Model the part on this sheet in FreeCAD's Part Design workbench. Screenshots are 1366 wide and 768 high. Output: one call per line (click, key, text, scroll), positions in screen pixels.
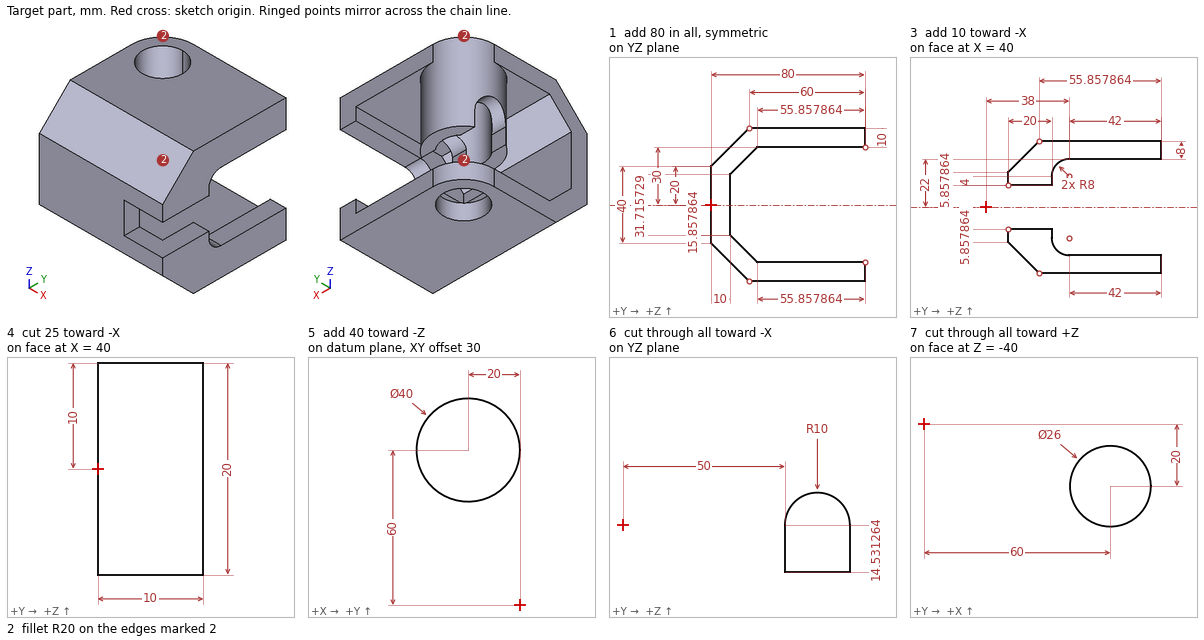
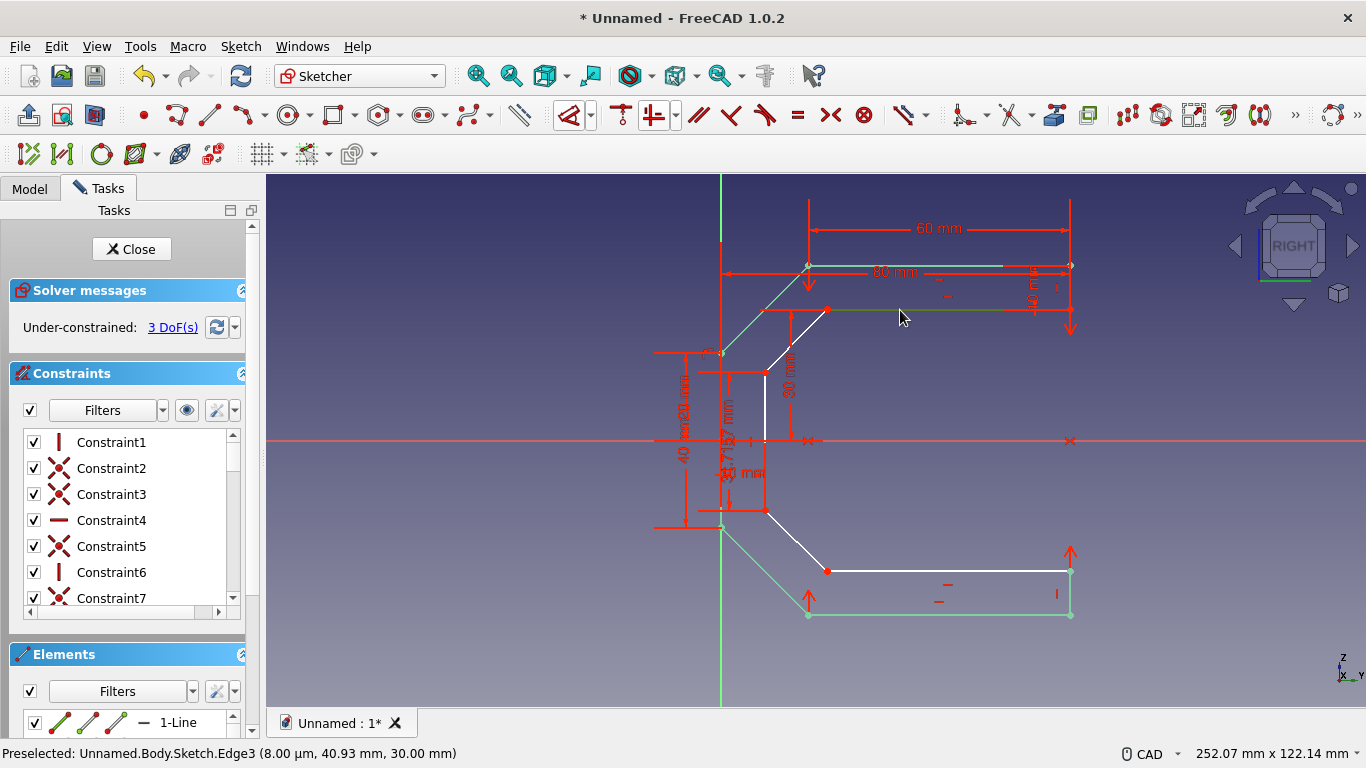
key(l)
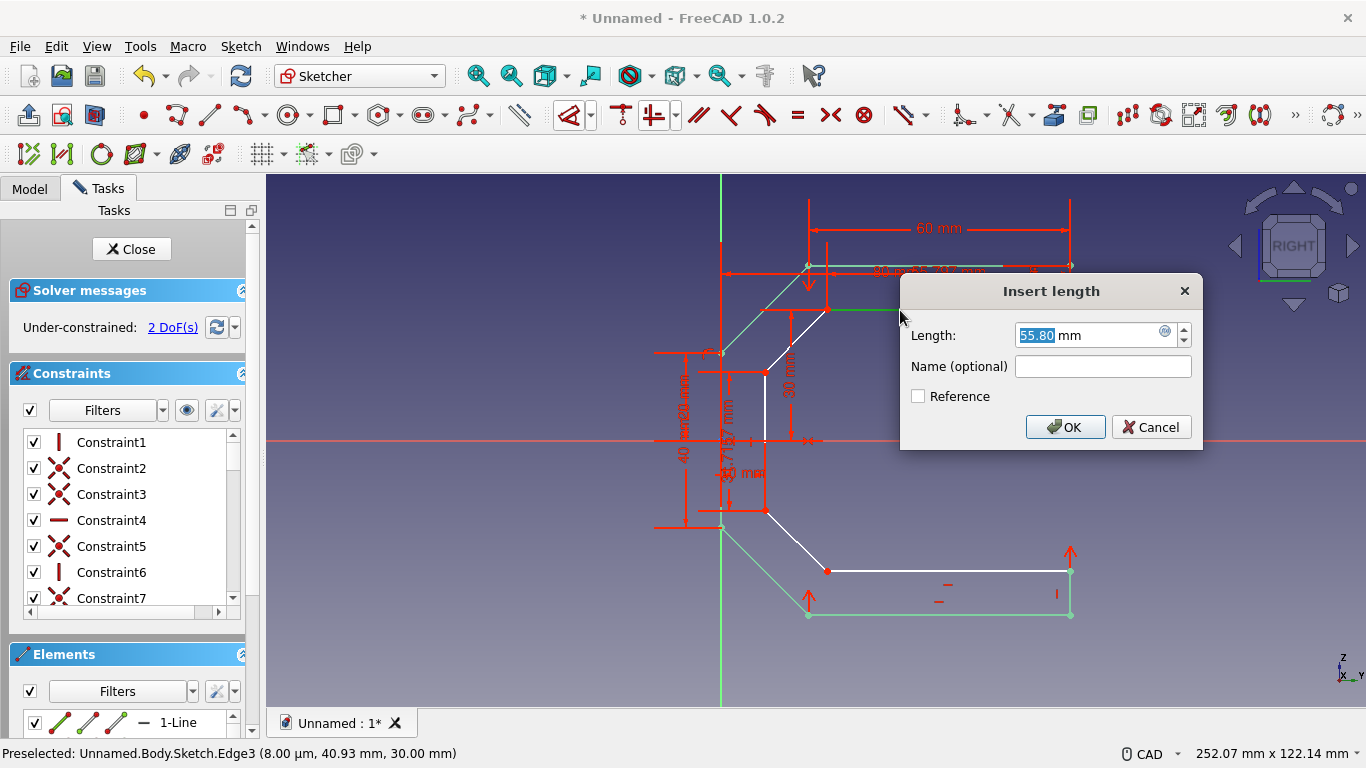
text(55.857864)
key(Return)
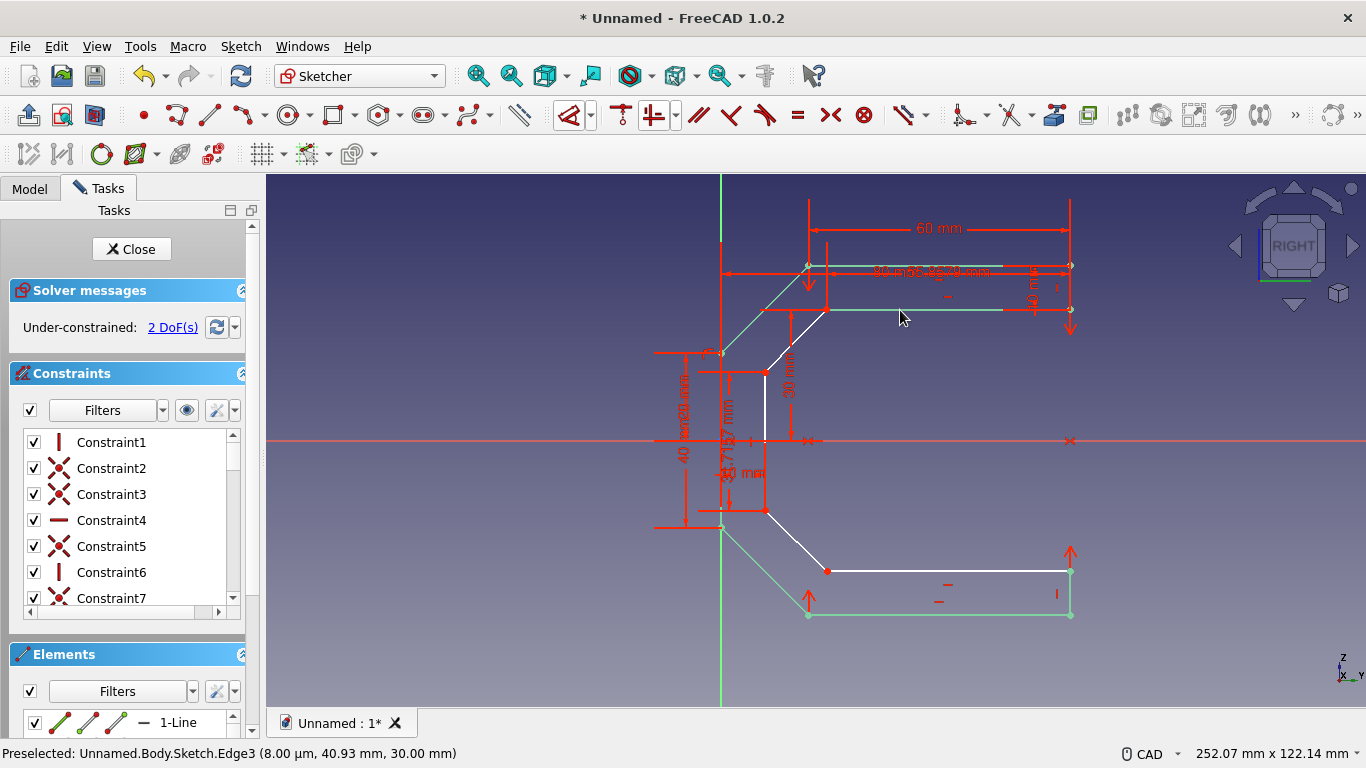
click(997, 571)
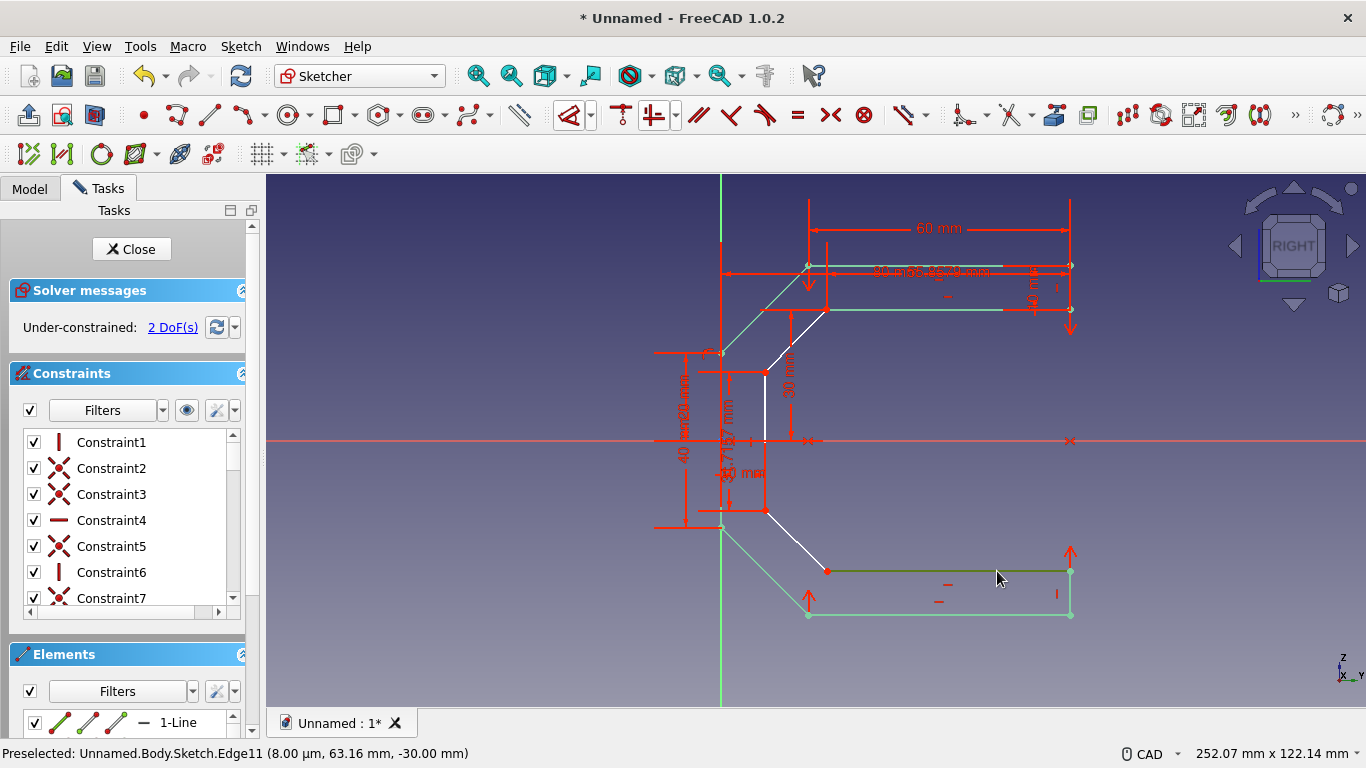
key(l)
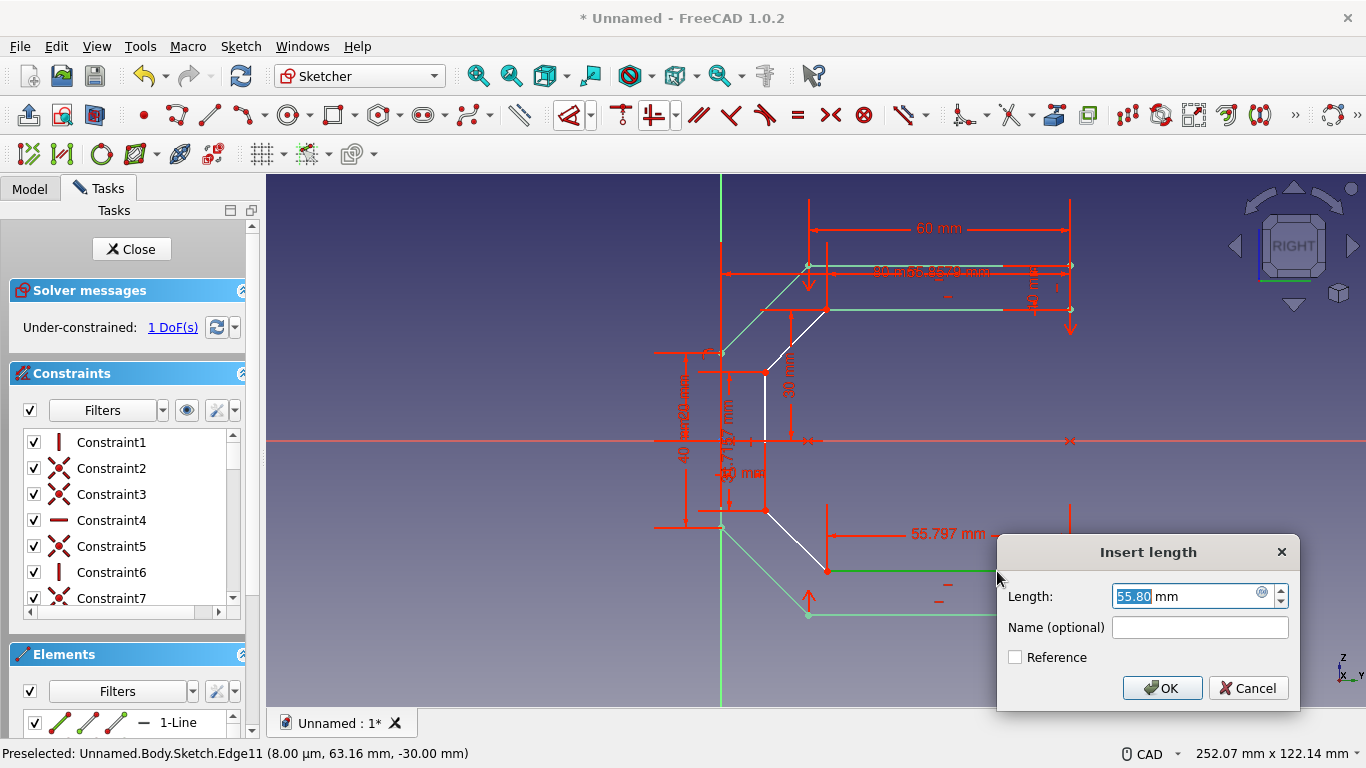
text(55.857864)
key(Return)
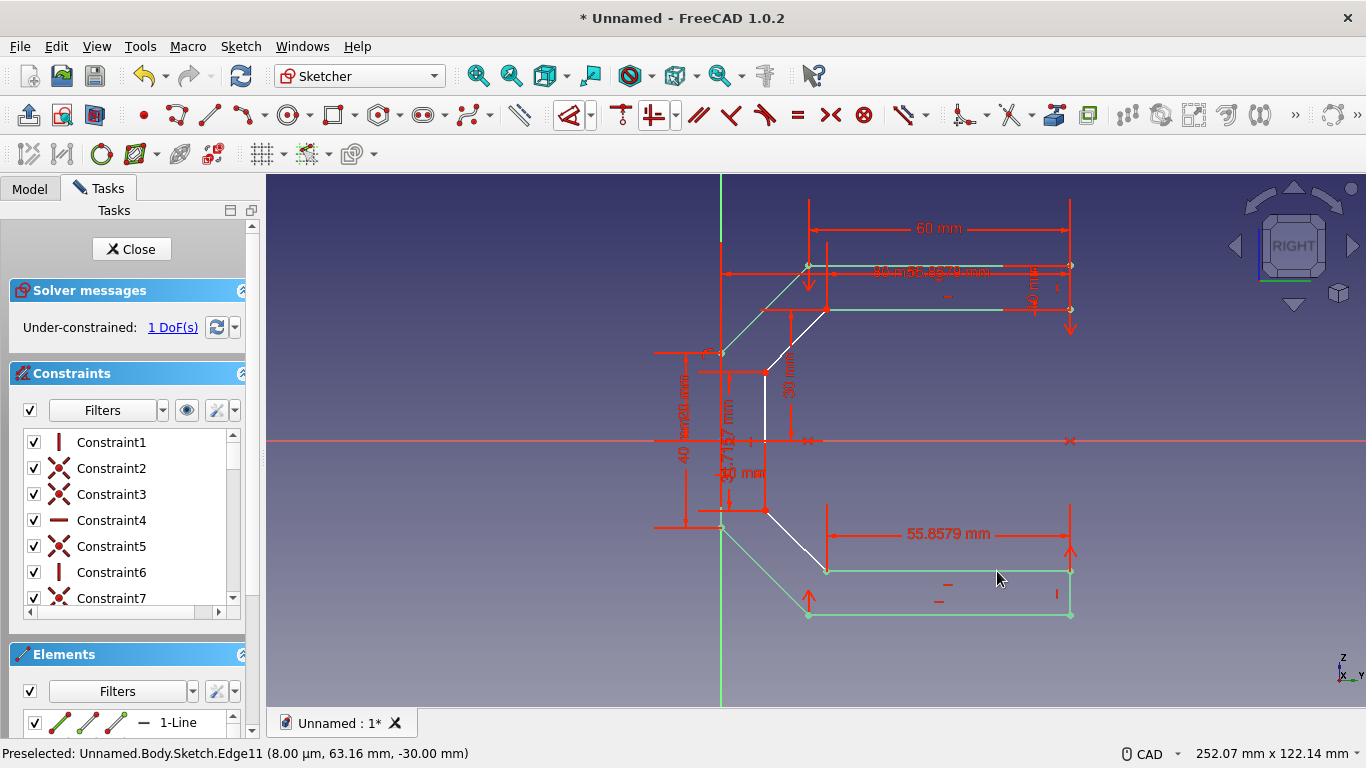
click(765, 511)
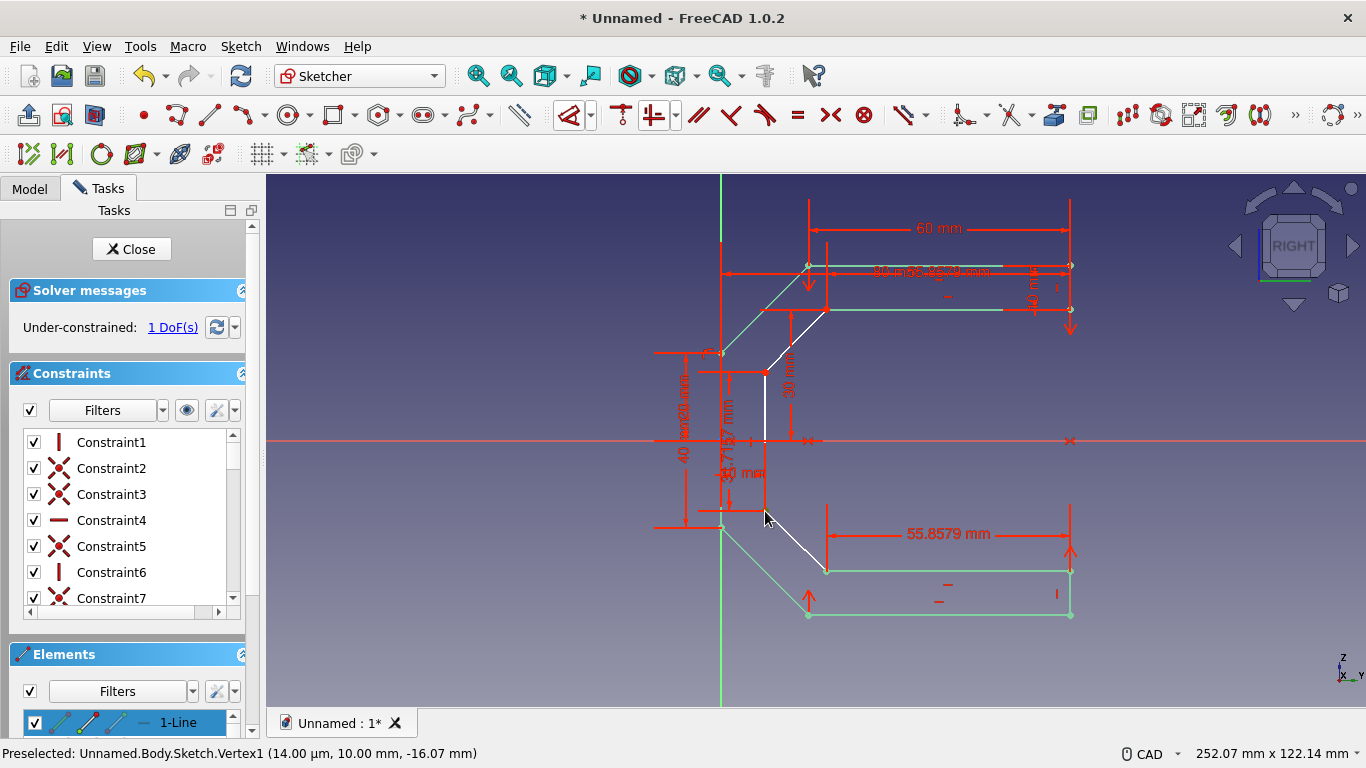
key(i)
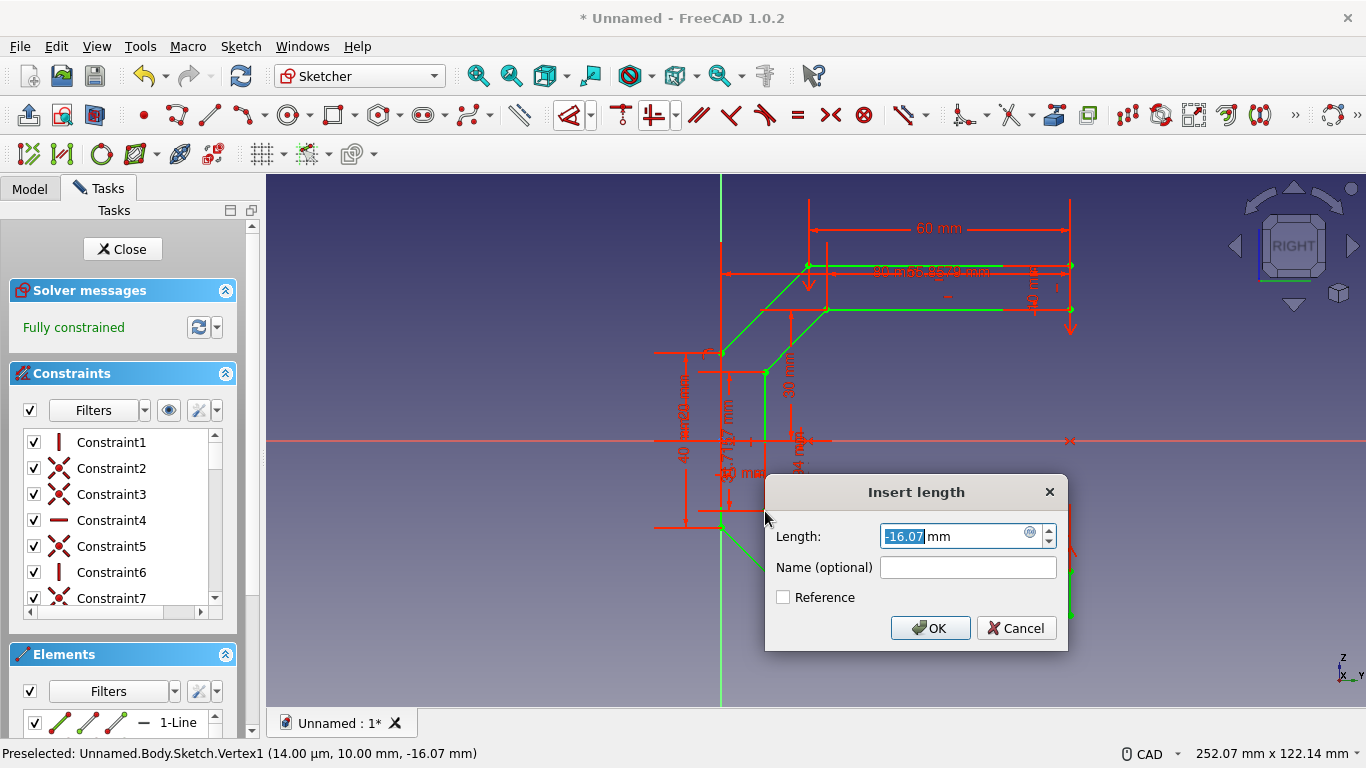
text(-15.857864)
key(Return)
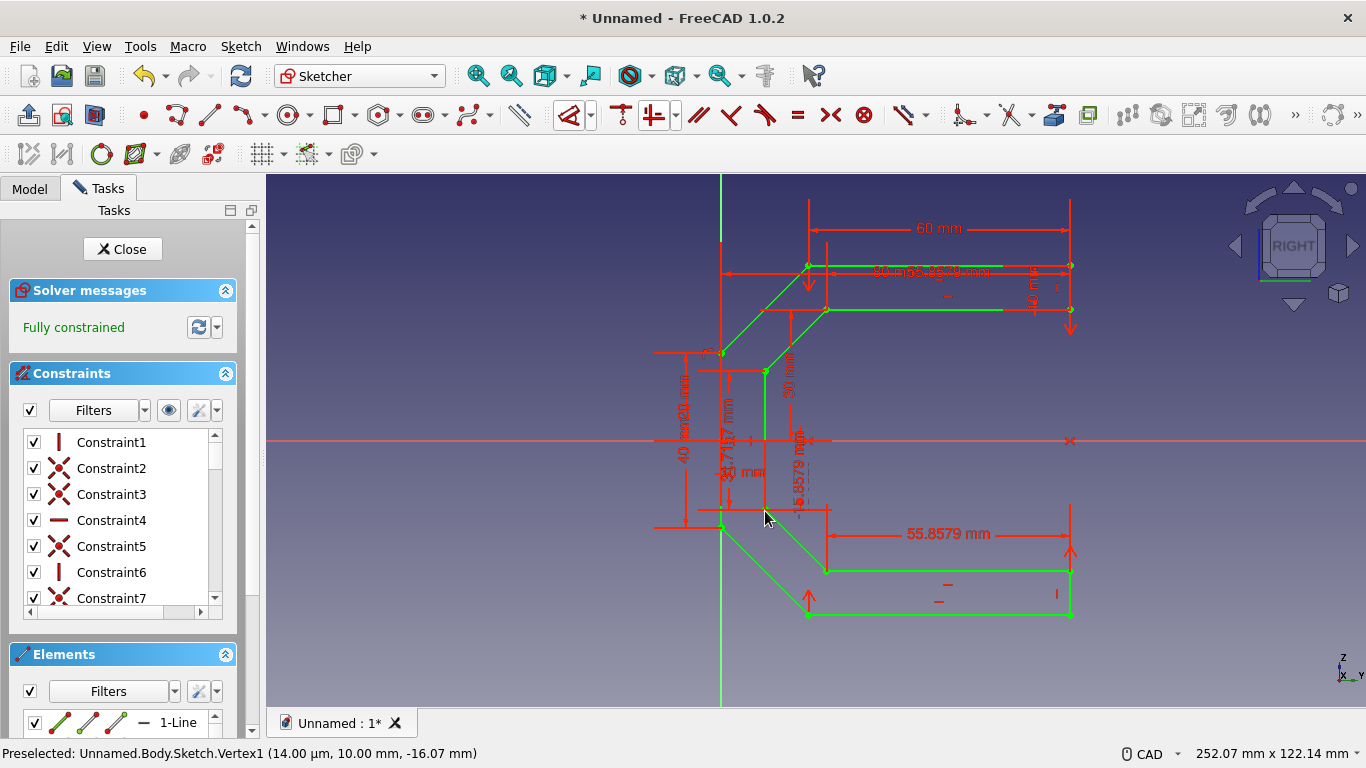
click(123, 249)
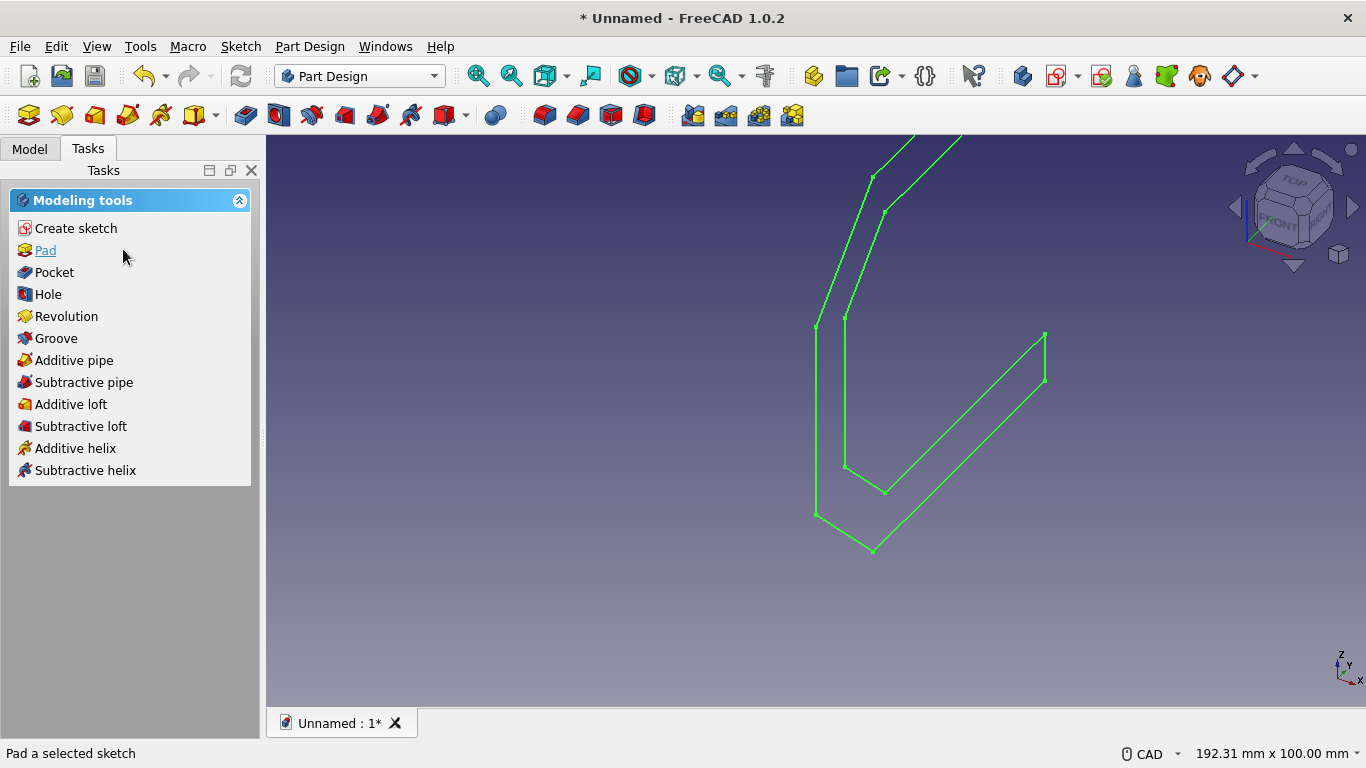
click(29, 116)